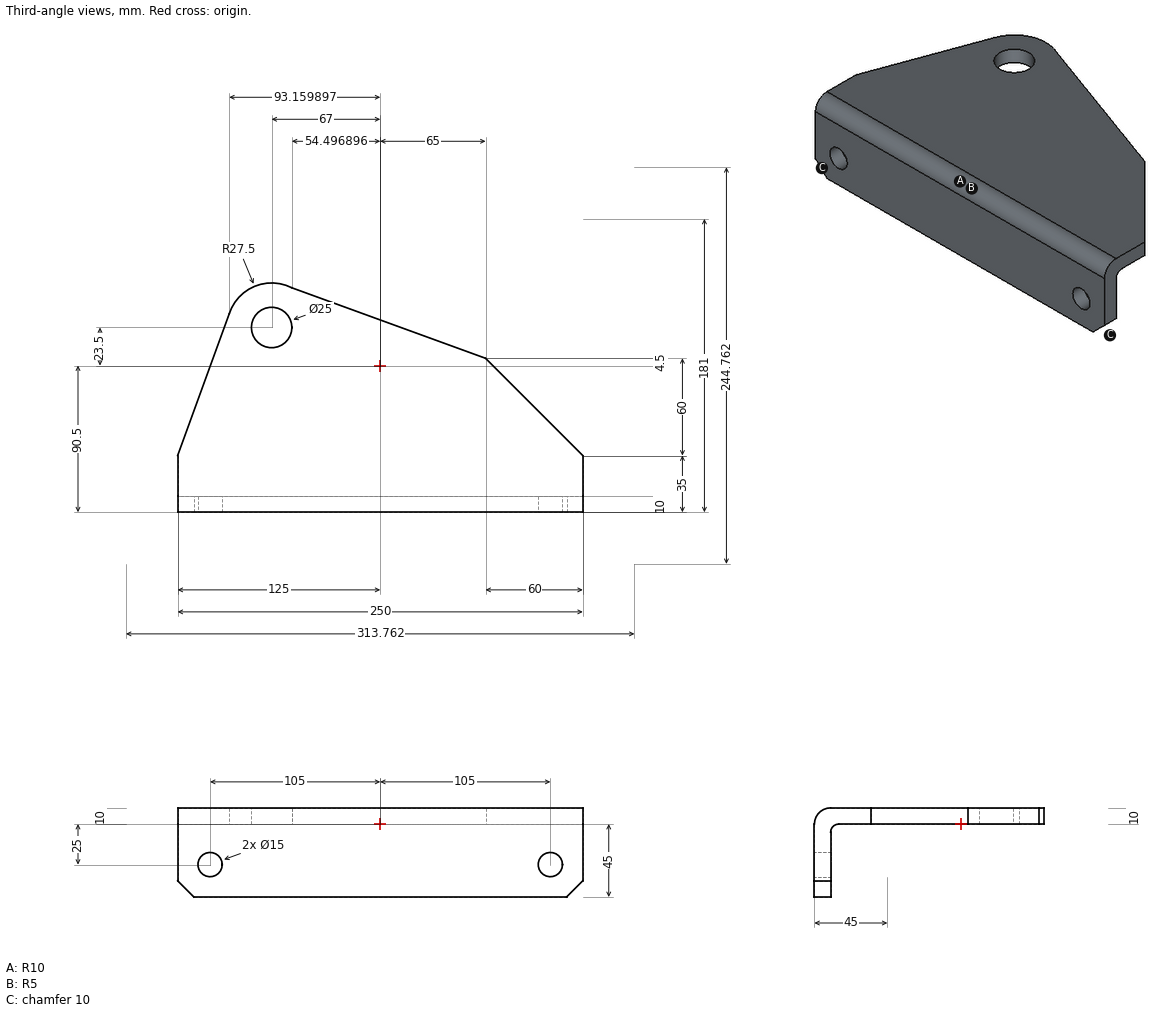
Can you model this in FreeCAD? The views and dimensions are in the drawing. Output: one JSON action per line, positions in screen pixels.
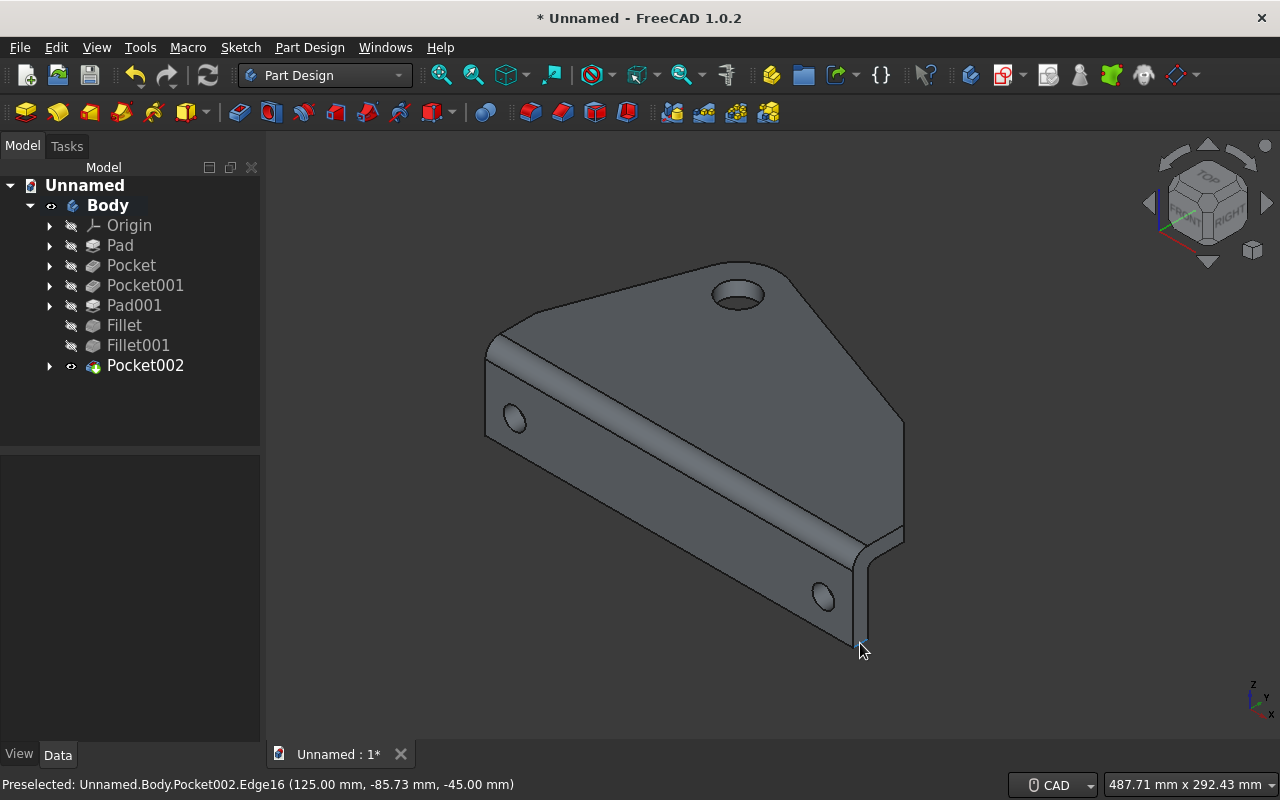
{"action": "key", "text": "2"}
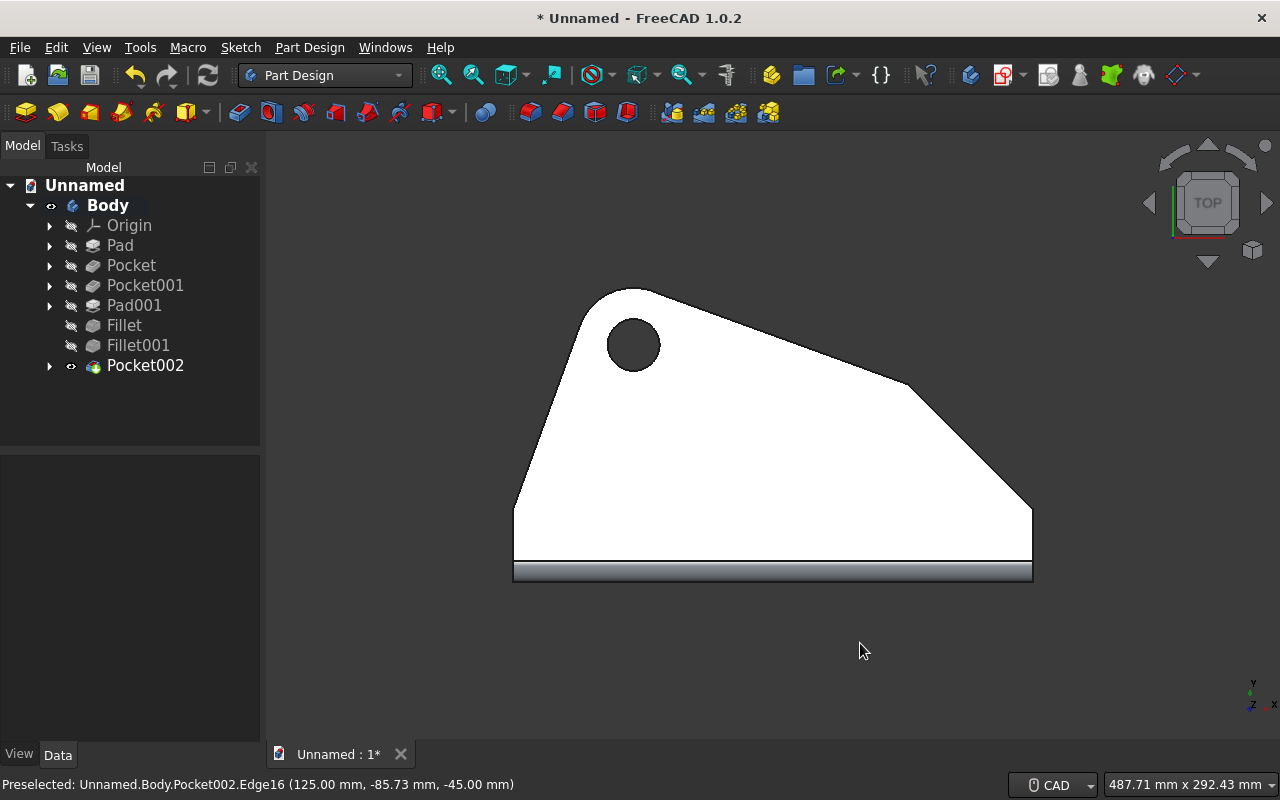
{"action": "scroll", "coordinate": [1033, 571], "scroll_direction": "up", "scroll_amount": 4}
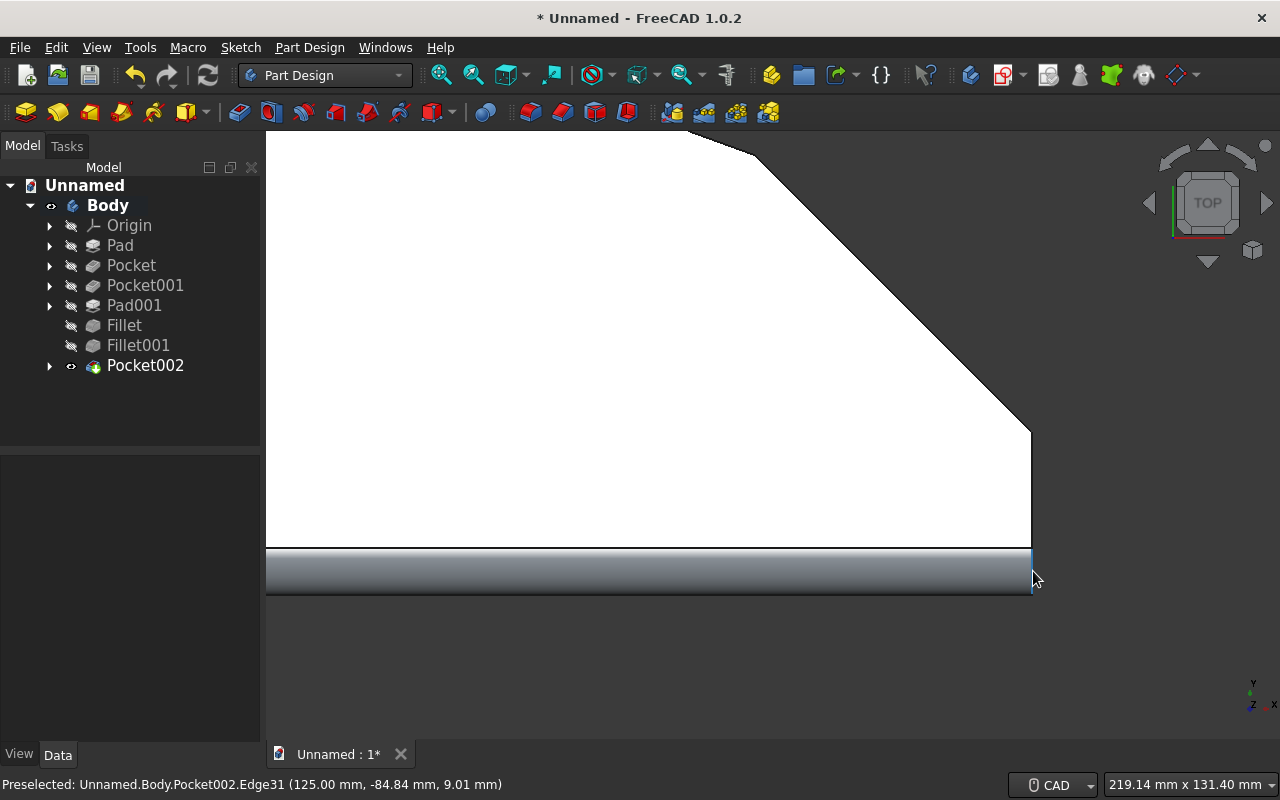
{"action": "key", "text": "v f"}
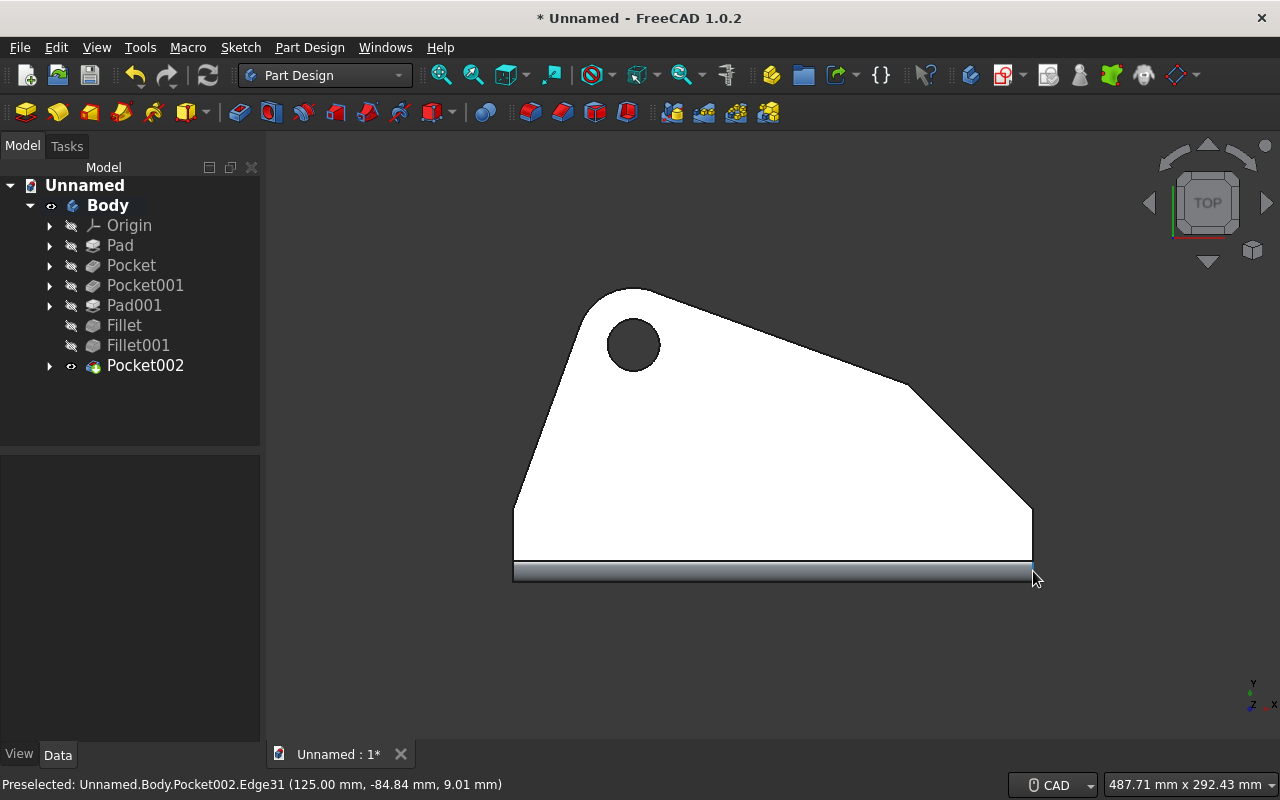
{"action": "key", "text": "0"}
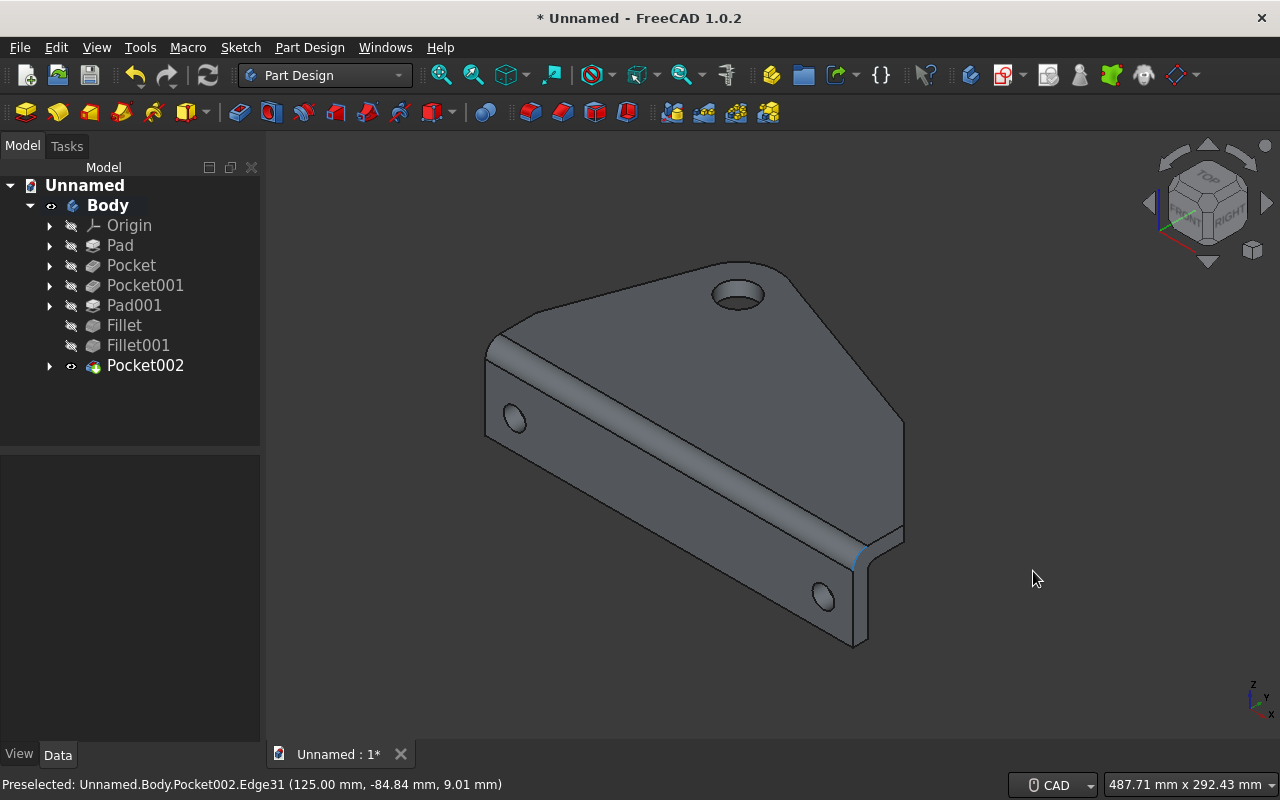
{"action": "scroll", "coordinate": [860, 643], "scroll_direction": "up", "scroll_amount": 4}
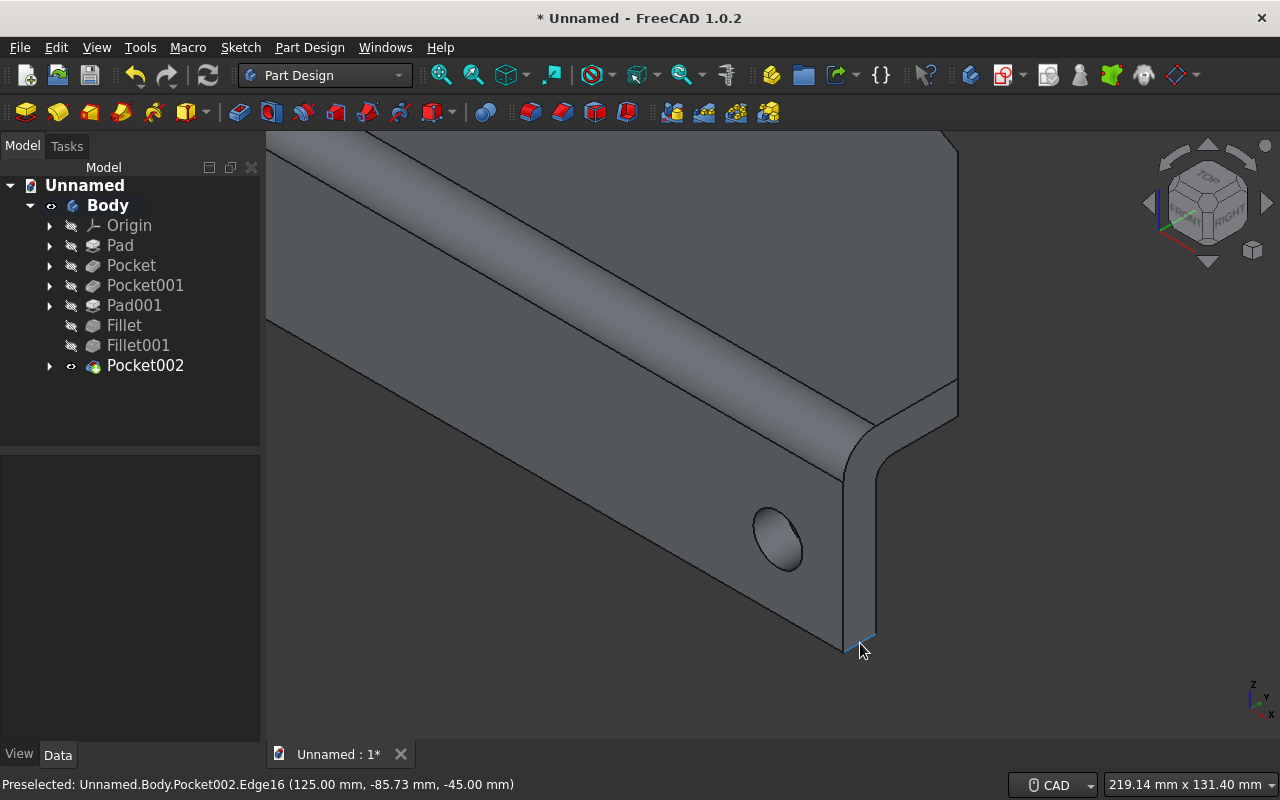
{"action": "left_click", "coordinate": [442, 76]}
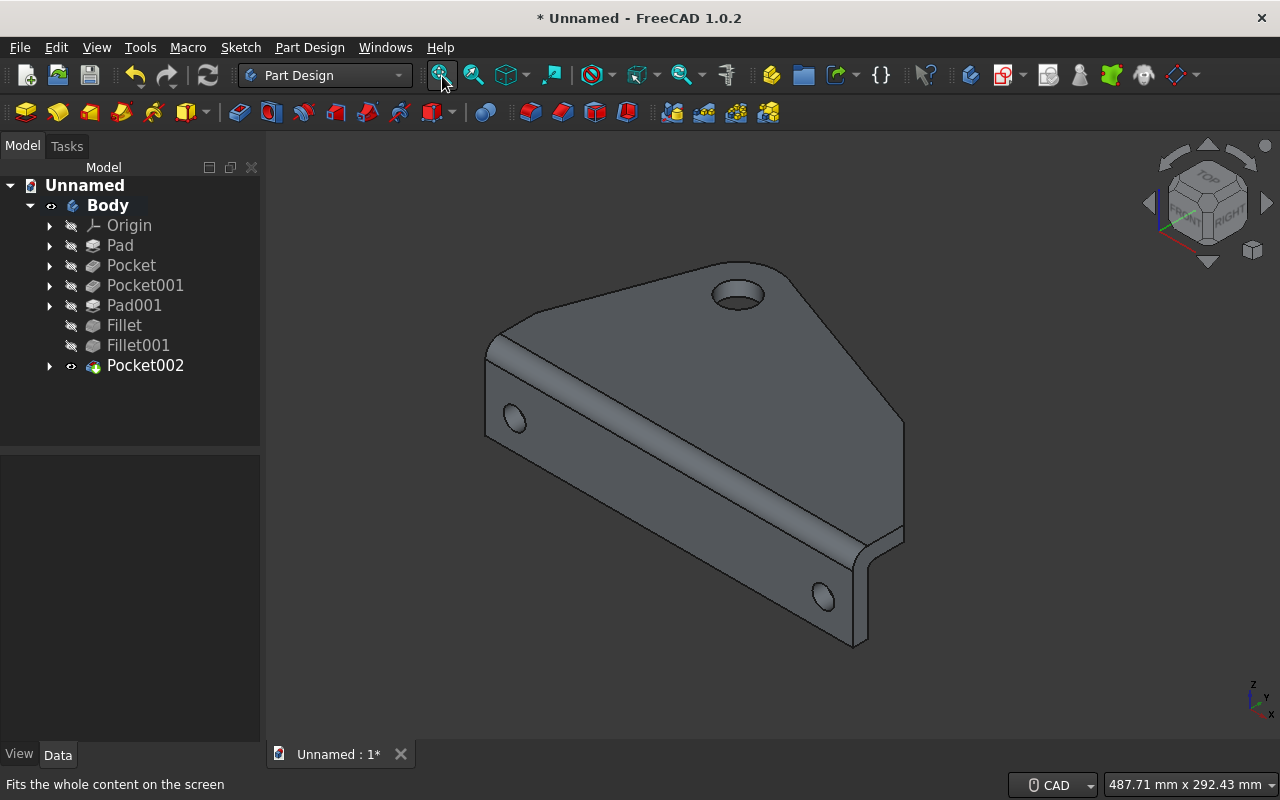
{"action": "key", "text": "1"}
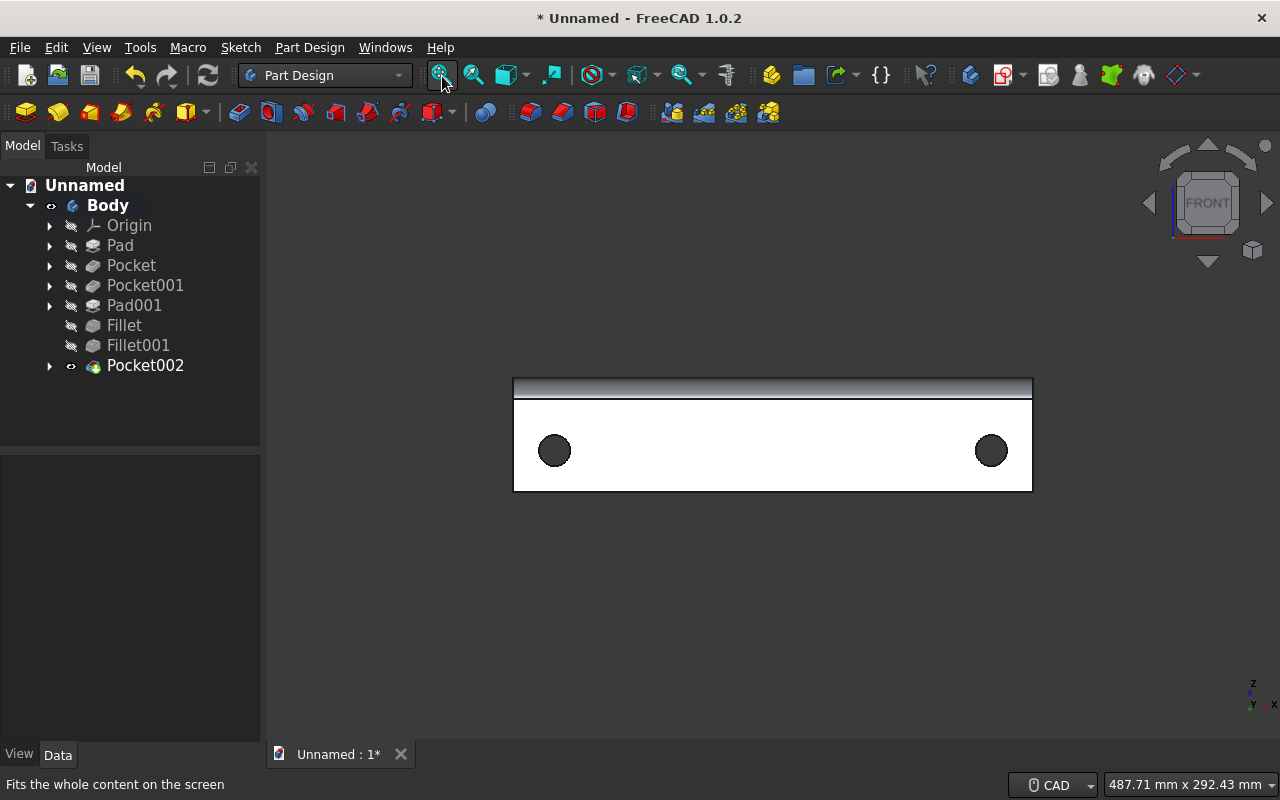
{"action": "scroll", "coordinate": [1033, 491], "scroll_direction": "up", "scroll_amount": 4}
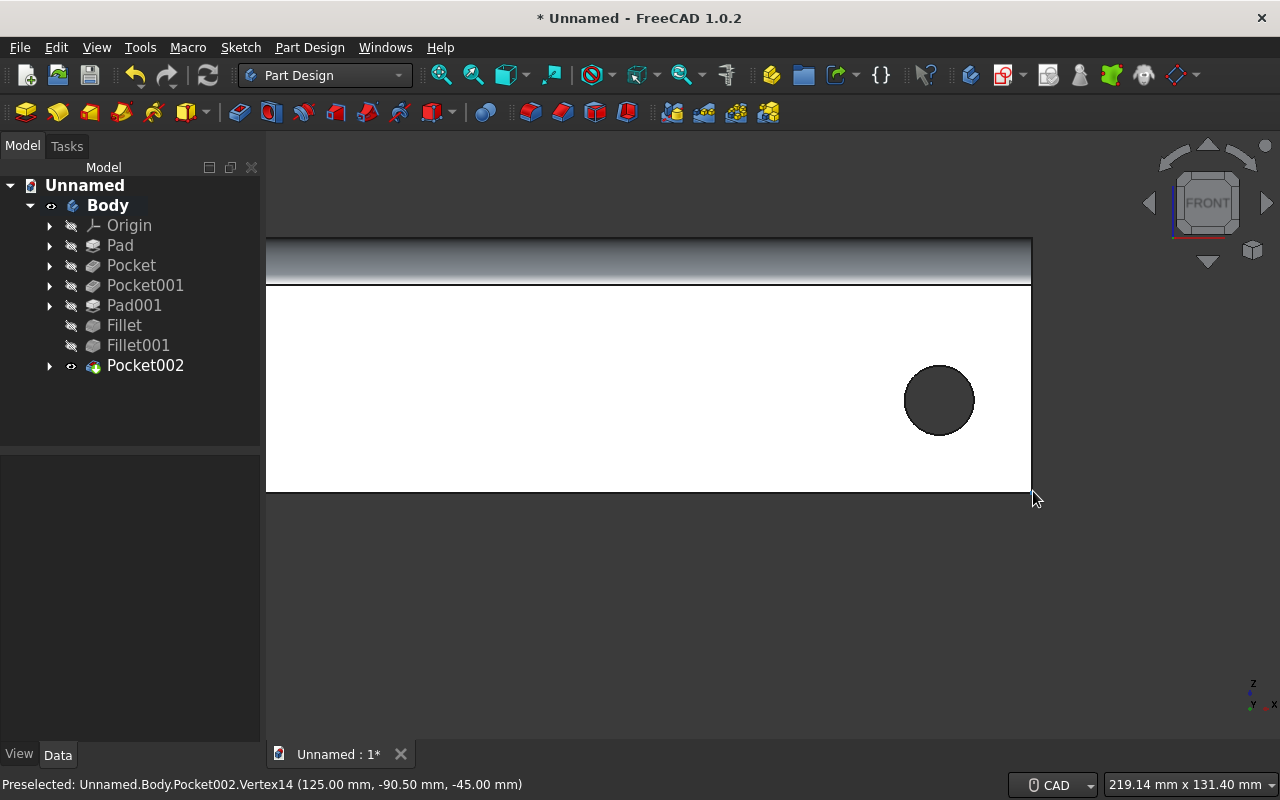
{"action": "left_click", "coordinate": [442, 76]}